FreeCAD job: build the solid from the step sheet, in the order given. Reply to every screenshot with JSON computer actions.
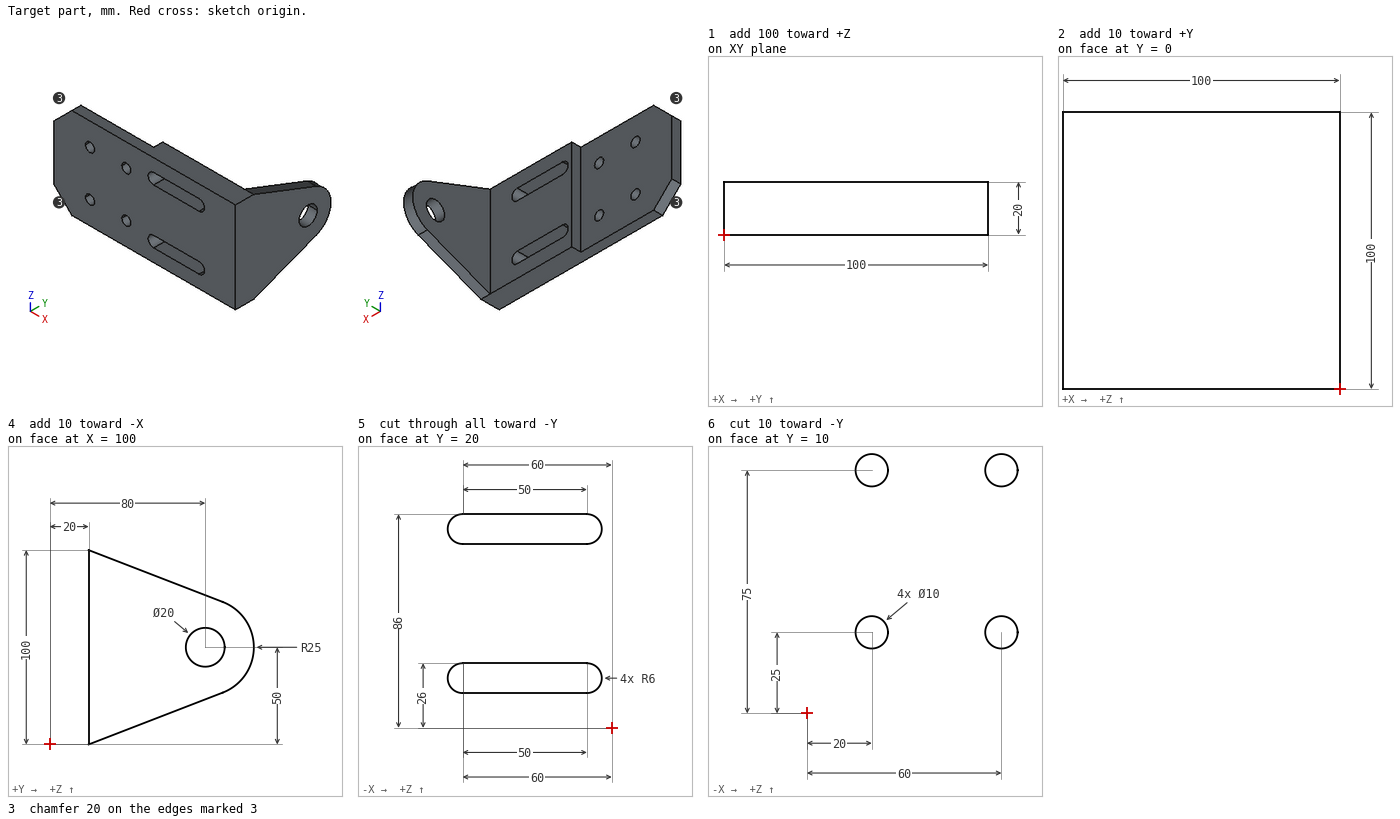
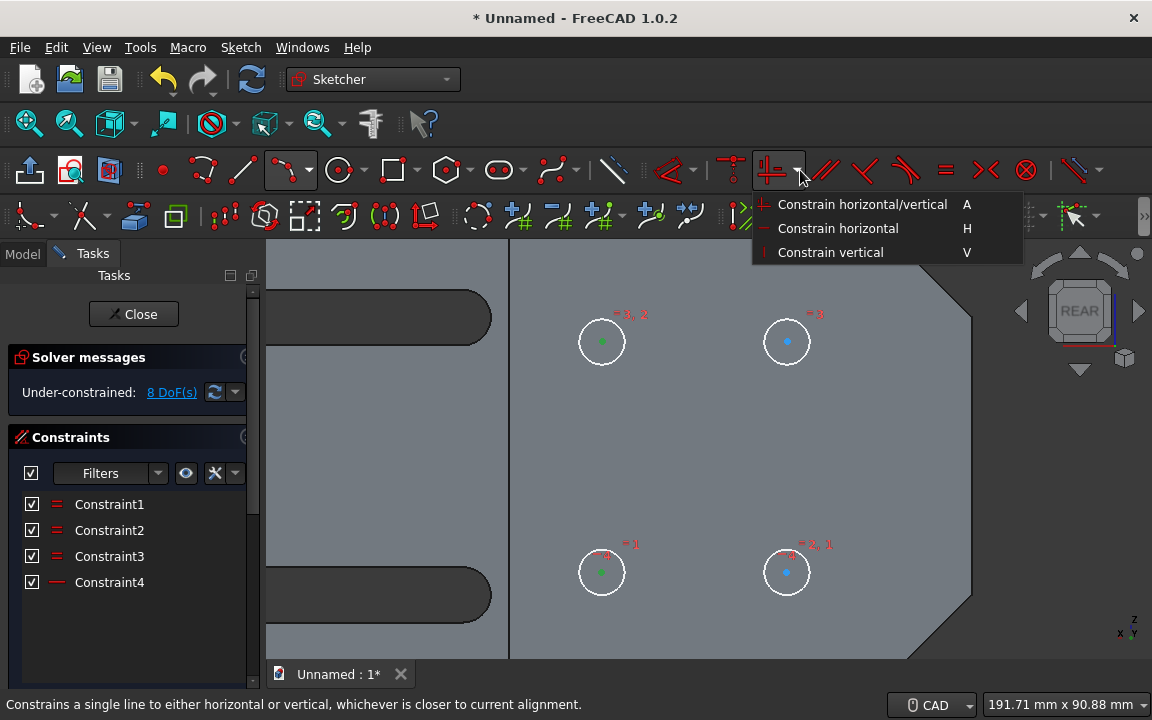
{"action": "left_click", "coordinate": [888, 252]}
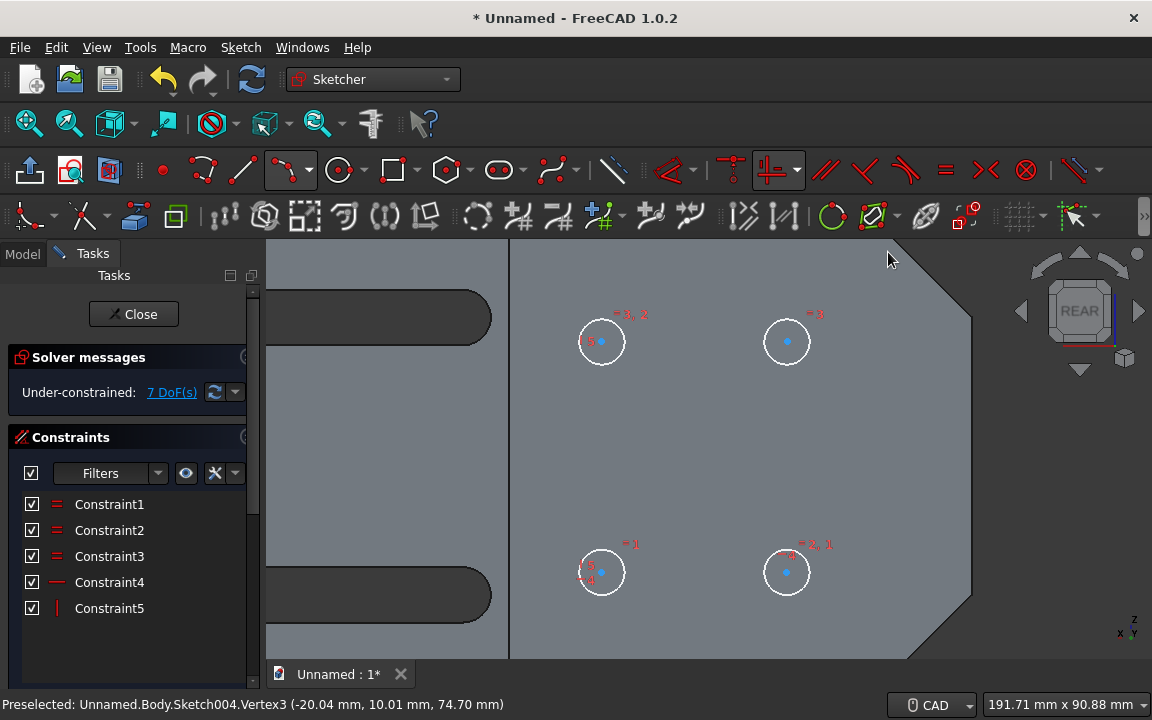
{"action": "left_click", "coordinate": [787, 572]}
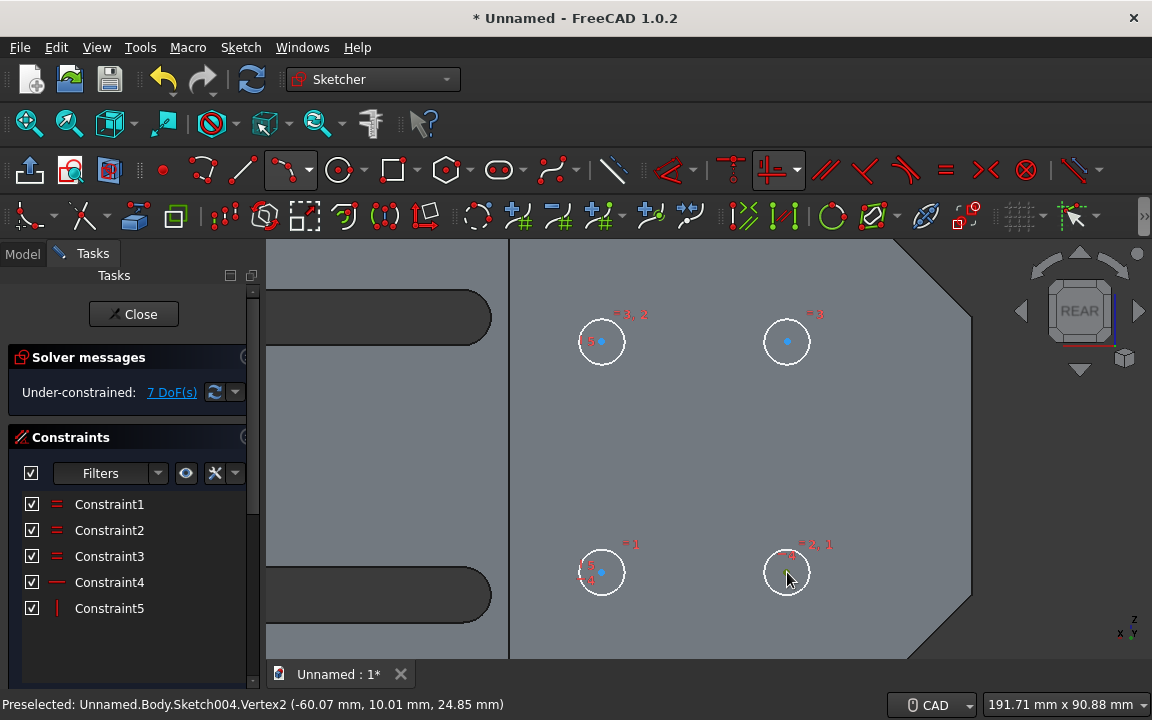
{"action": "left_click", "coordinate": [787, 342]}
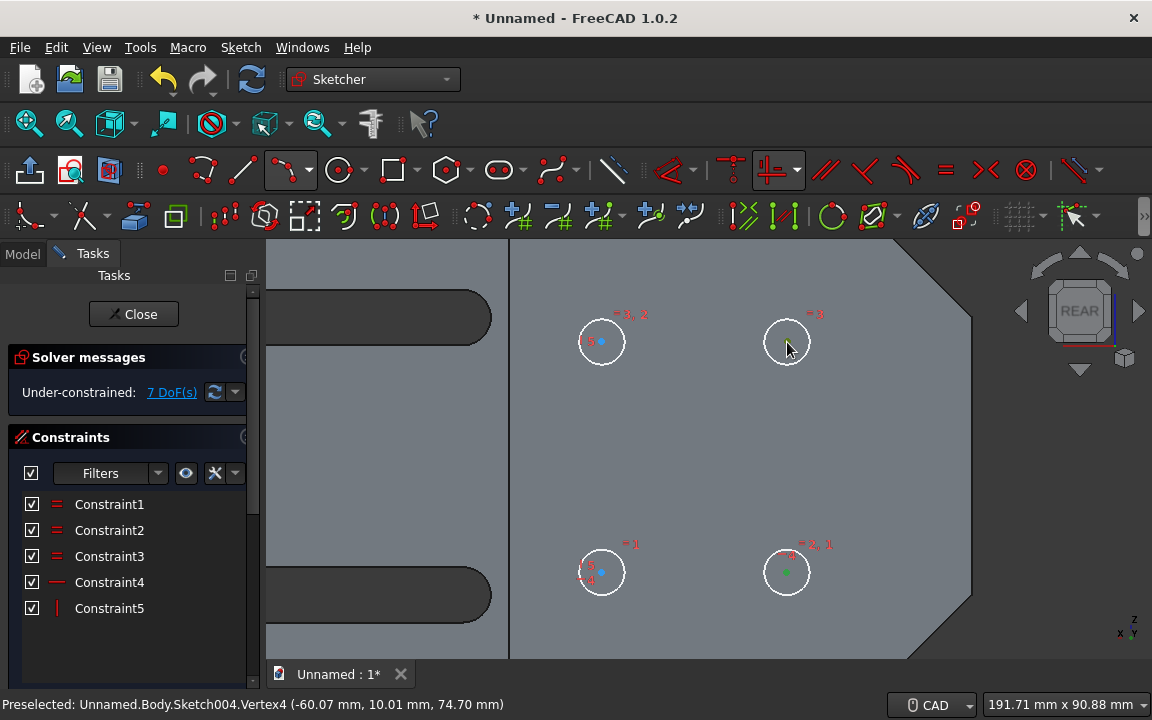
{"action": "left_click", "coordinate": [800, 170]}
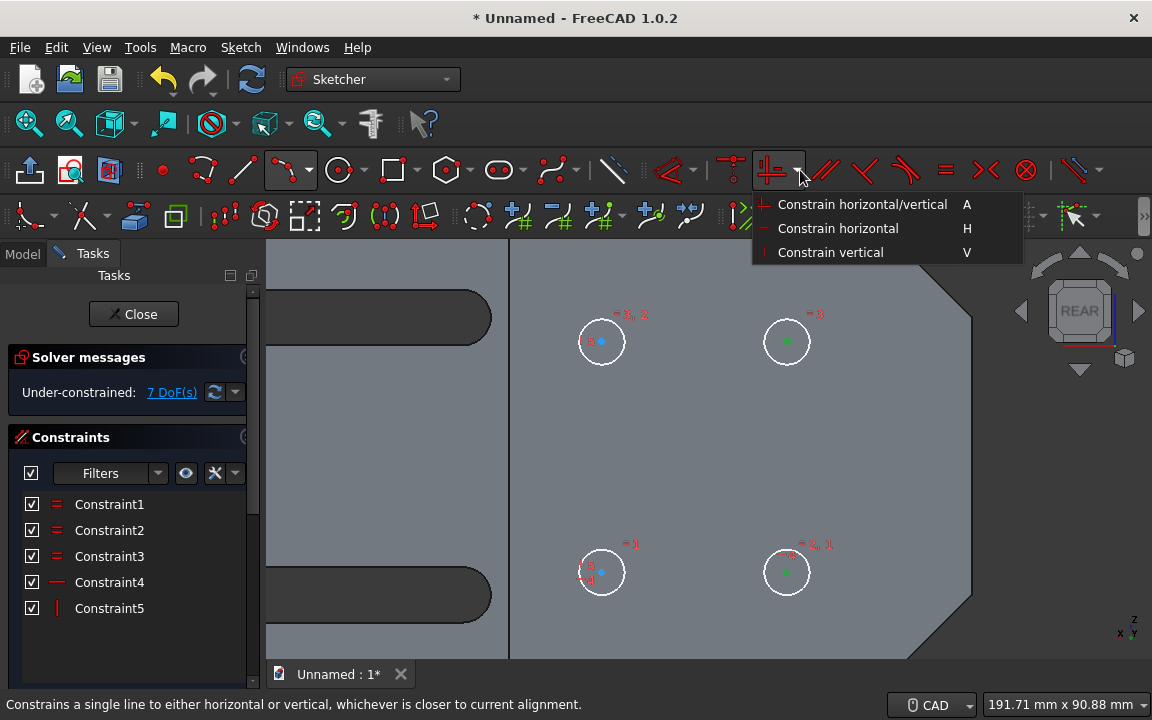
{"action": "left_click", "coordinate": [888, 252]}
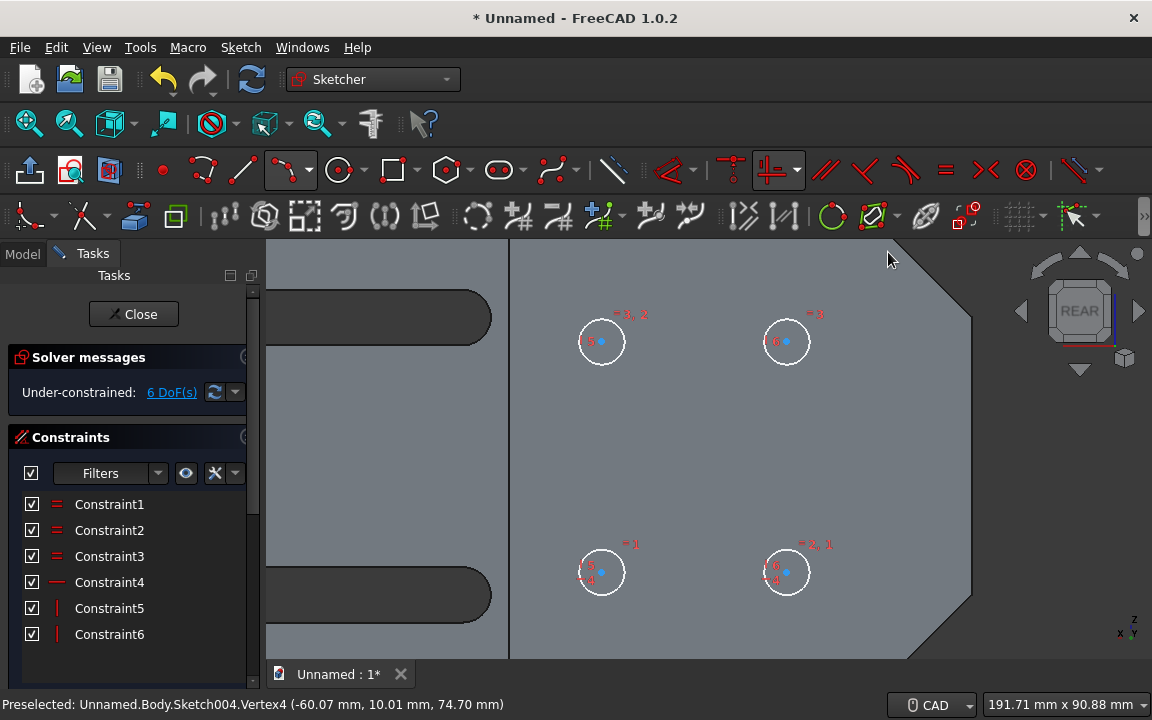
{"action": "left_click", "coordinate": [602, 342]}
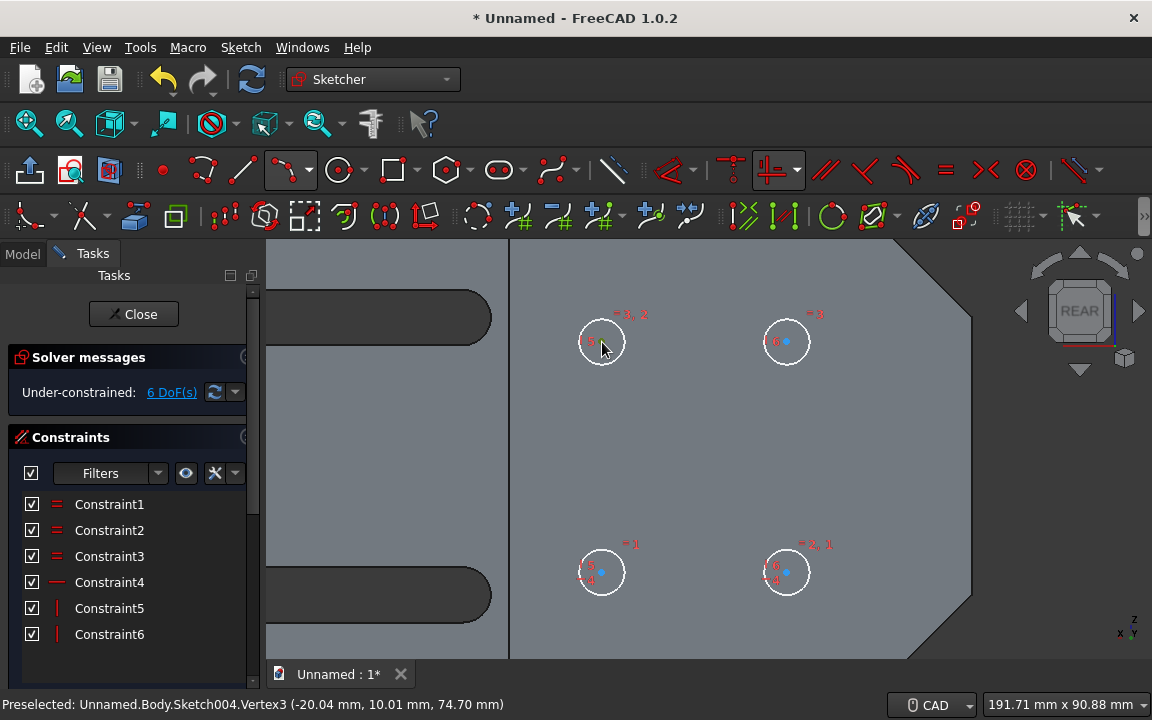
{"action": "left_click", "coordinate": [787, 342]}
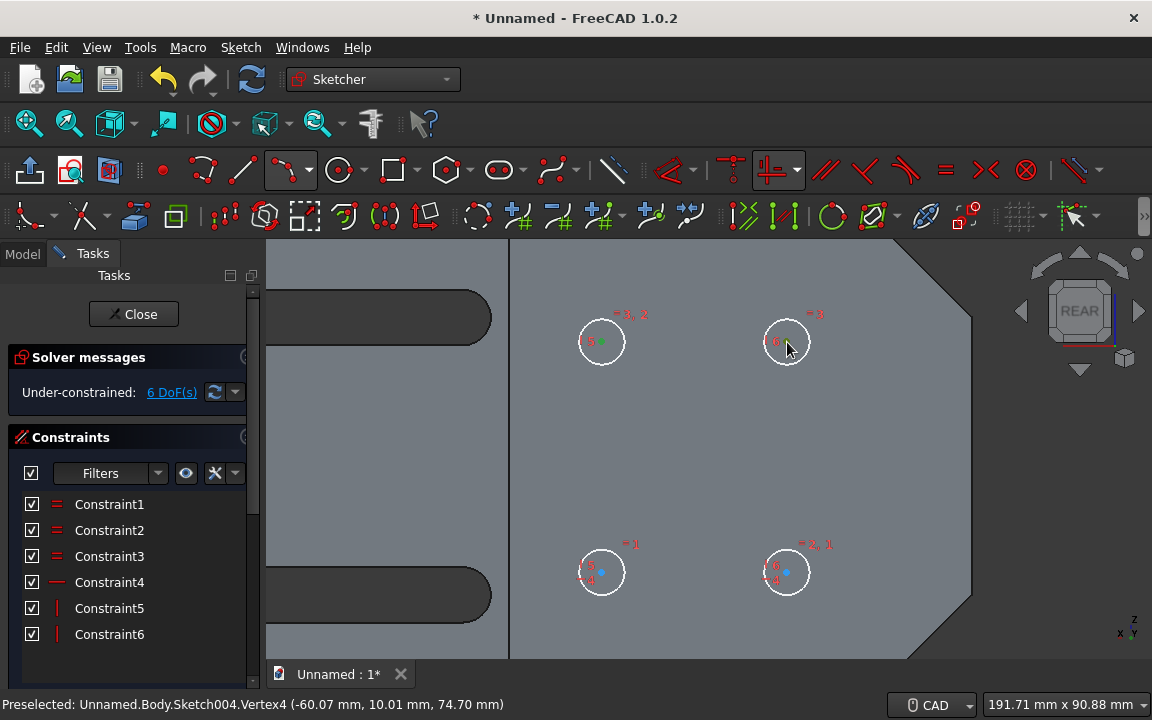
{"action": "left_click", "coordinate": [800, 170]}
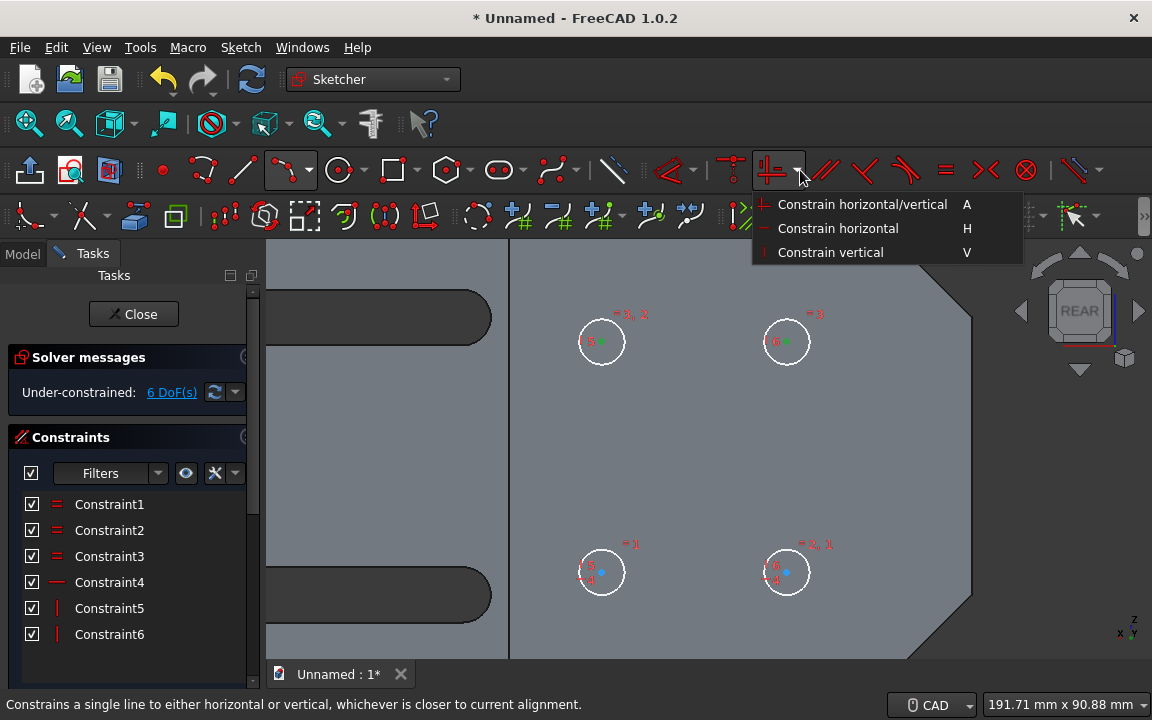
{"action": "left_click", "coordinate": [888, 228]}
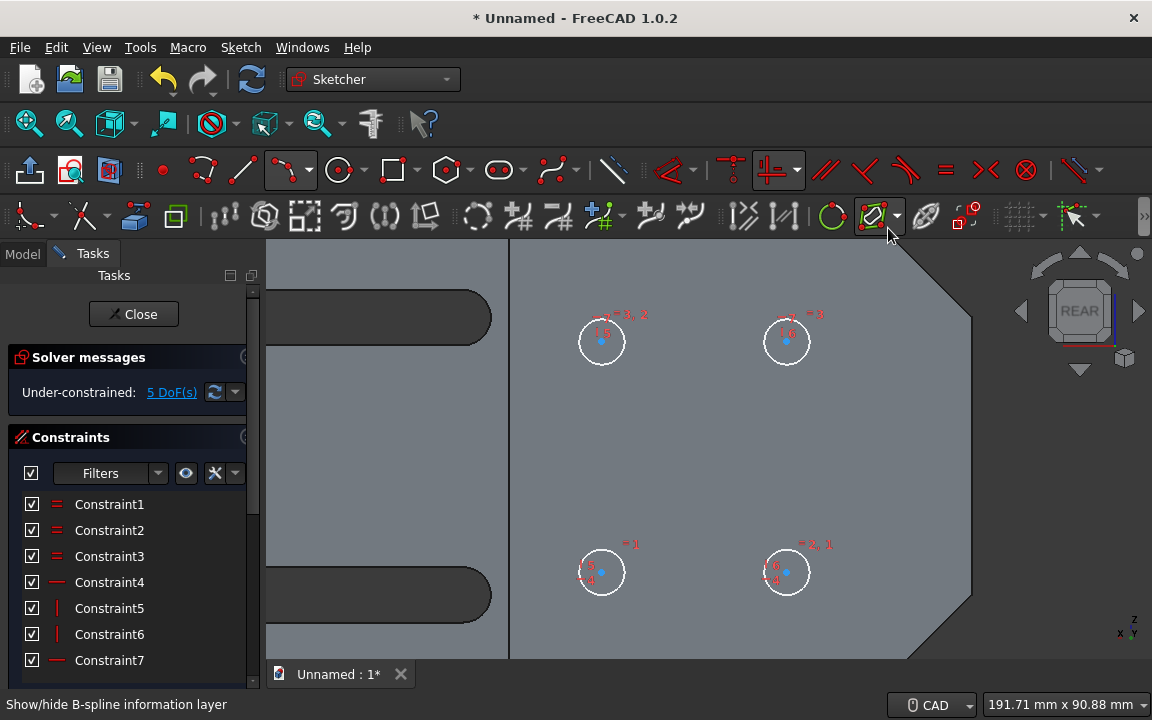
{"action": "left_click", "coordinate": [668, 170]}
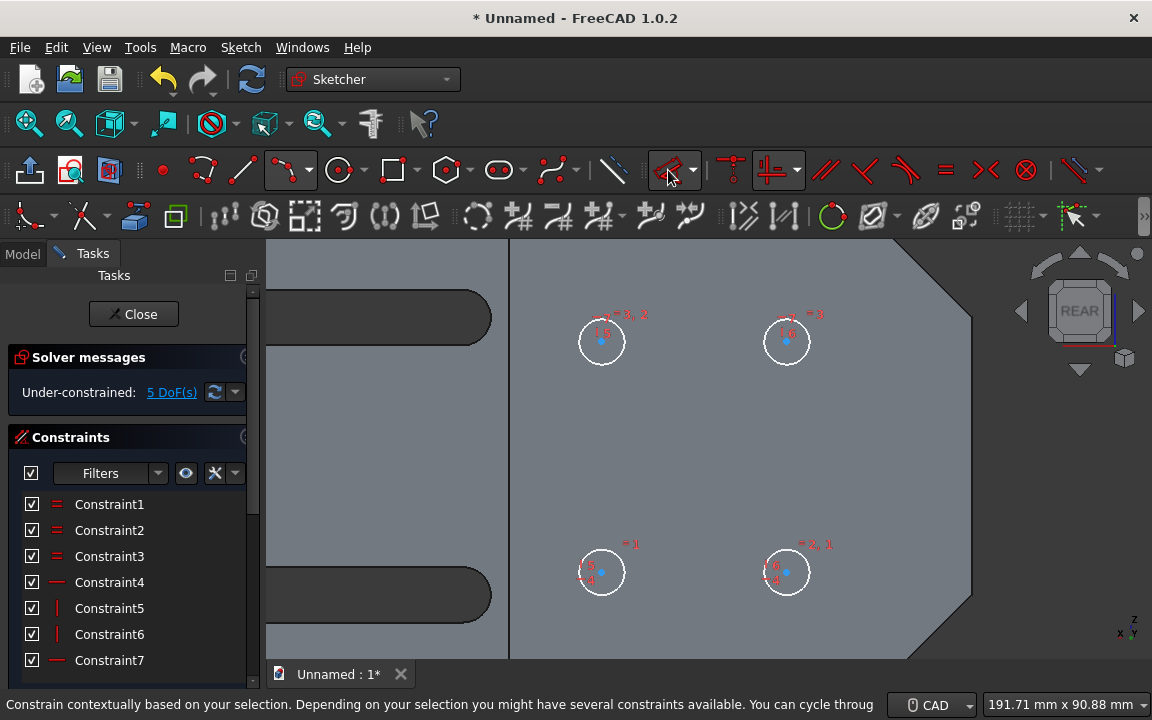
{"action": "left_click", "coordinate": [618, 556]}
{"action": "left_click", "coordinate": [640, 533]}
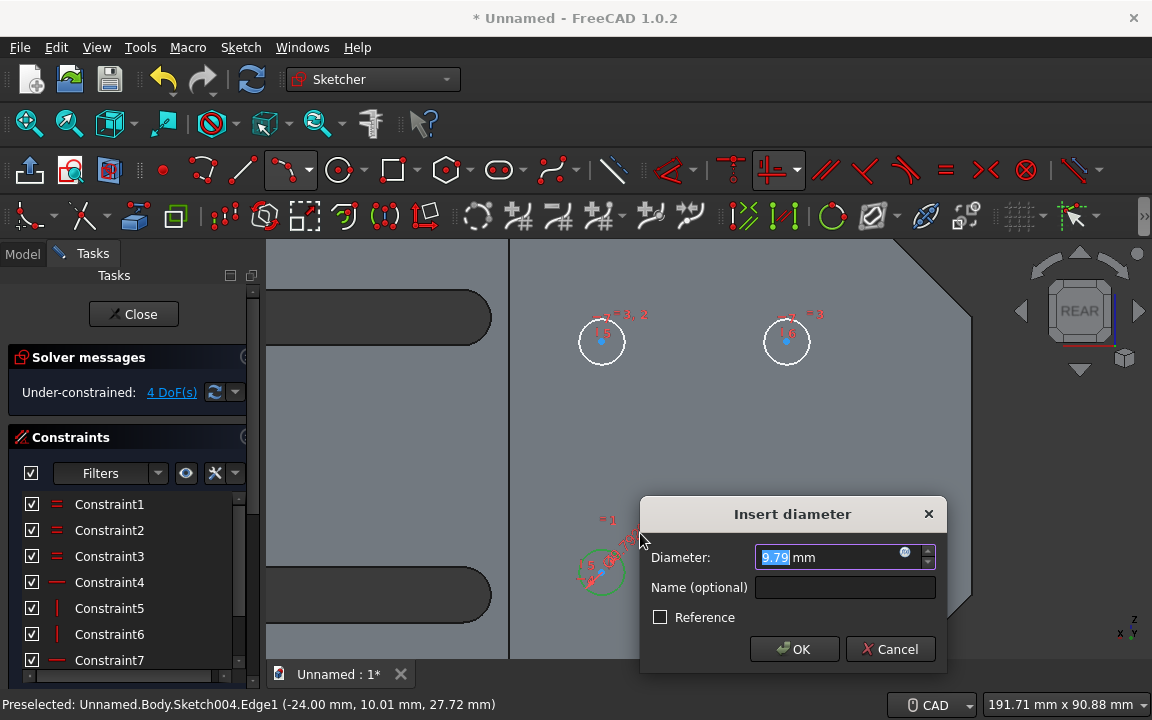
{"action": "type", "text": "10"}
{"action": "key", "text": "Return"}